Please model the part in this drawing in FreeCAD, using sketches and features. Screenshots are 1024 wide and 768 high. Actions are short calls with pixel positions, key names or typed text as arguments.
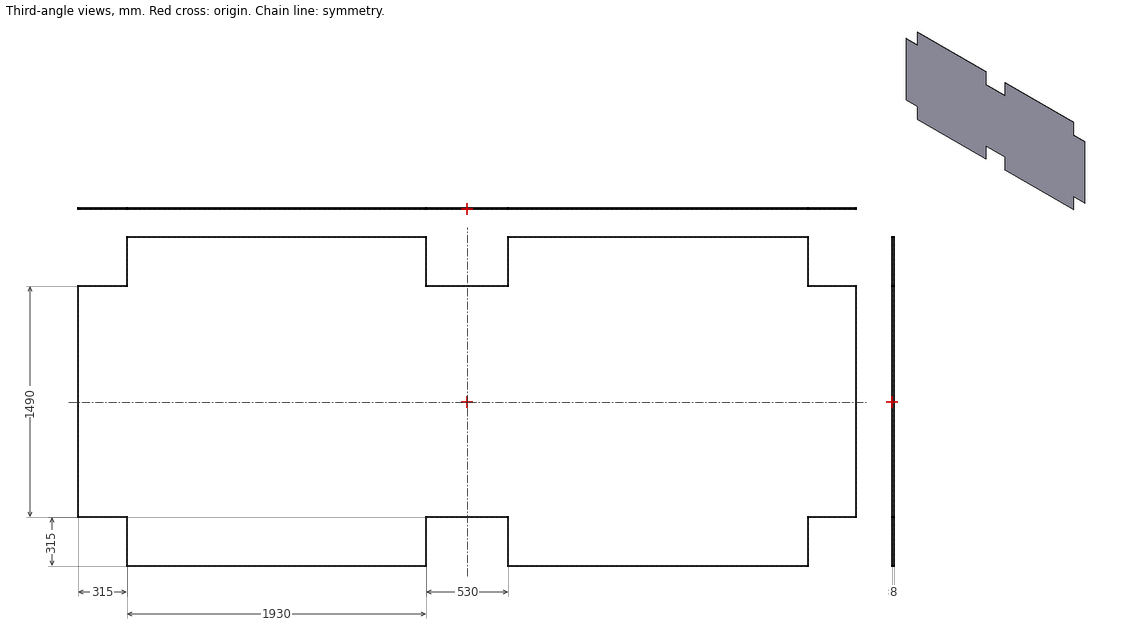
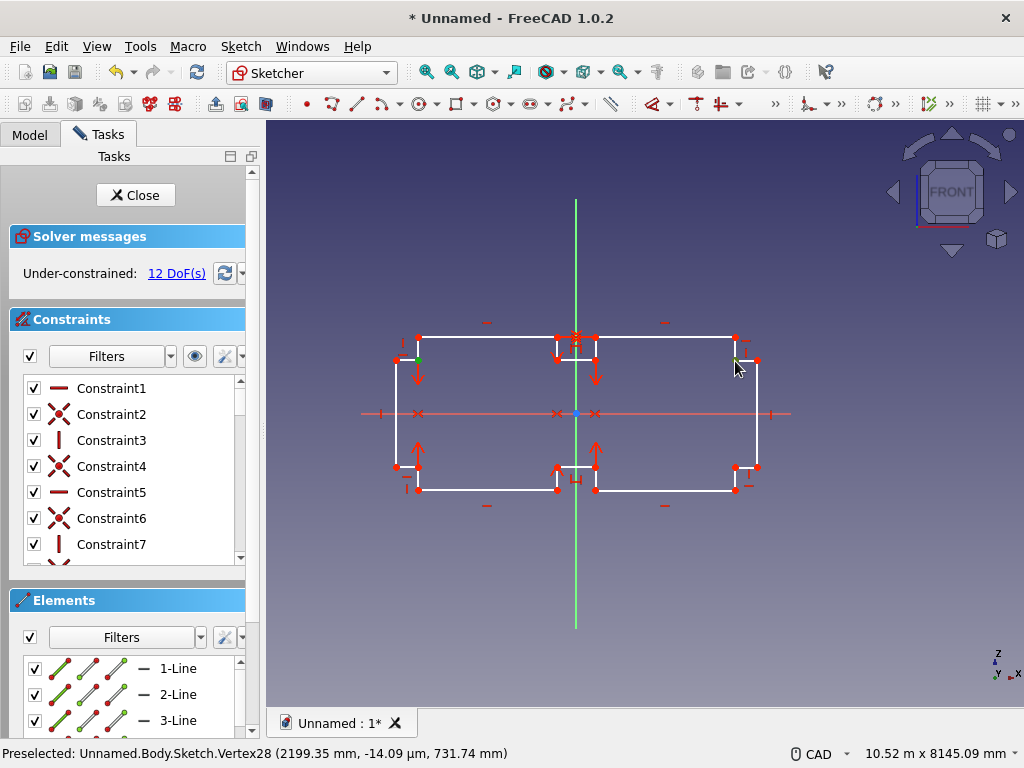
click(576, 603)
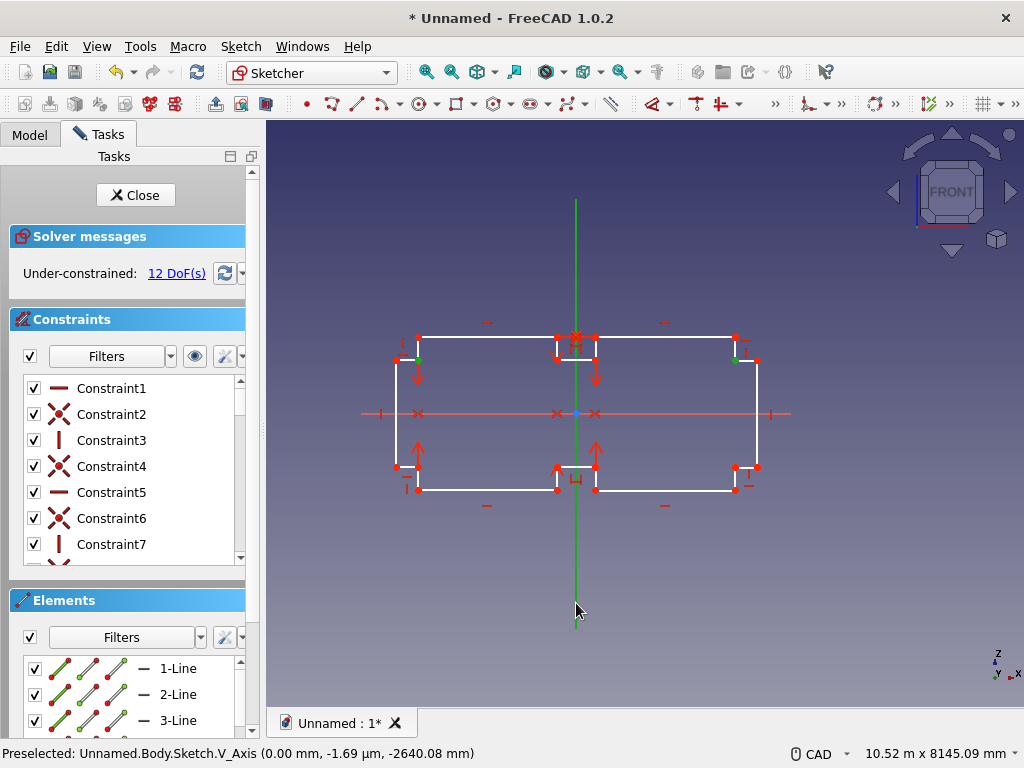
key(s)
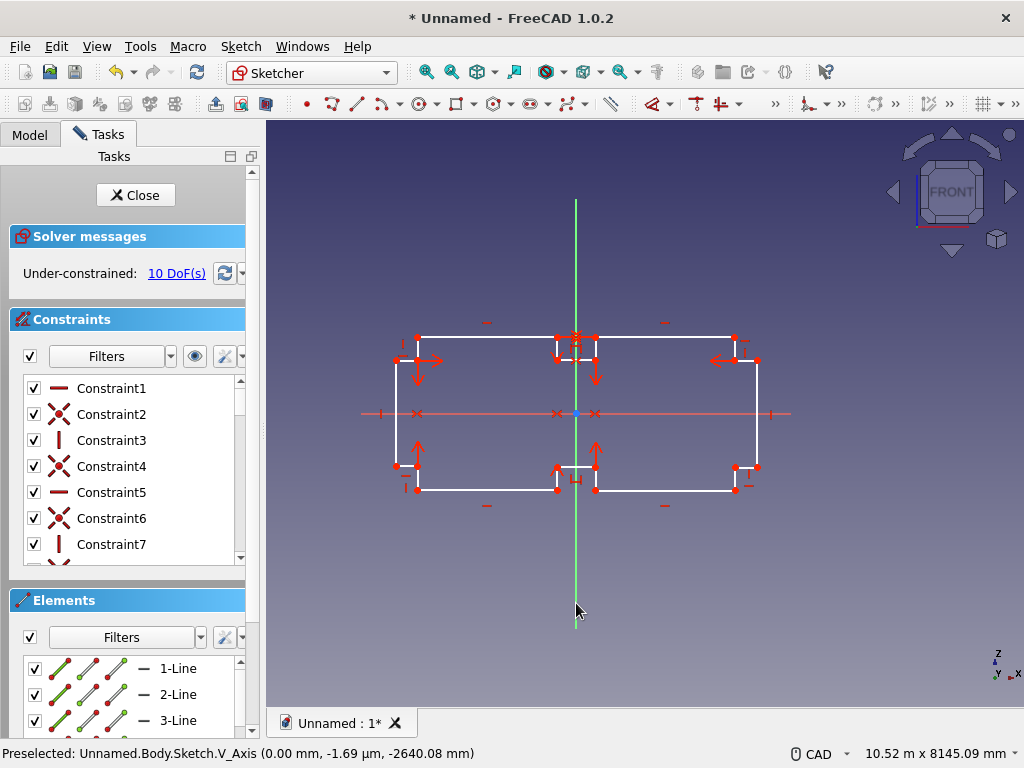
click(396, 466)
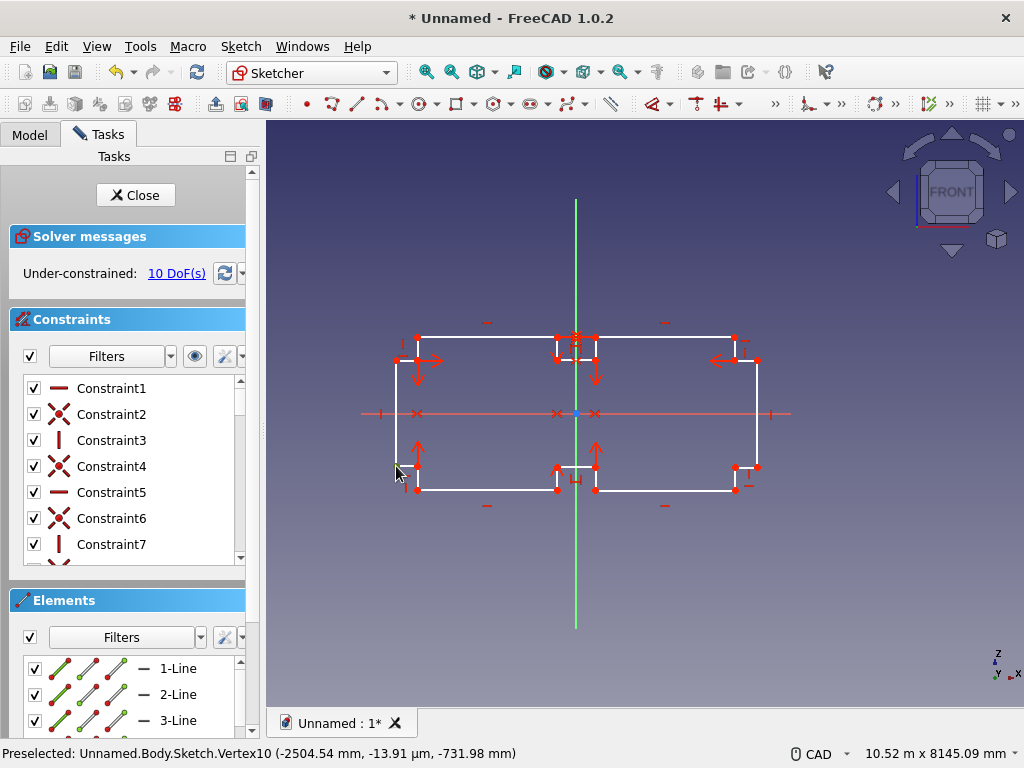
click(757, 468)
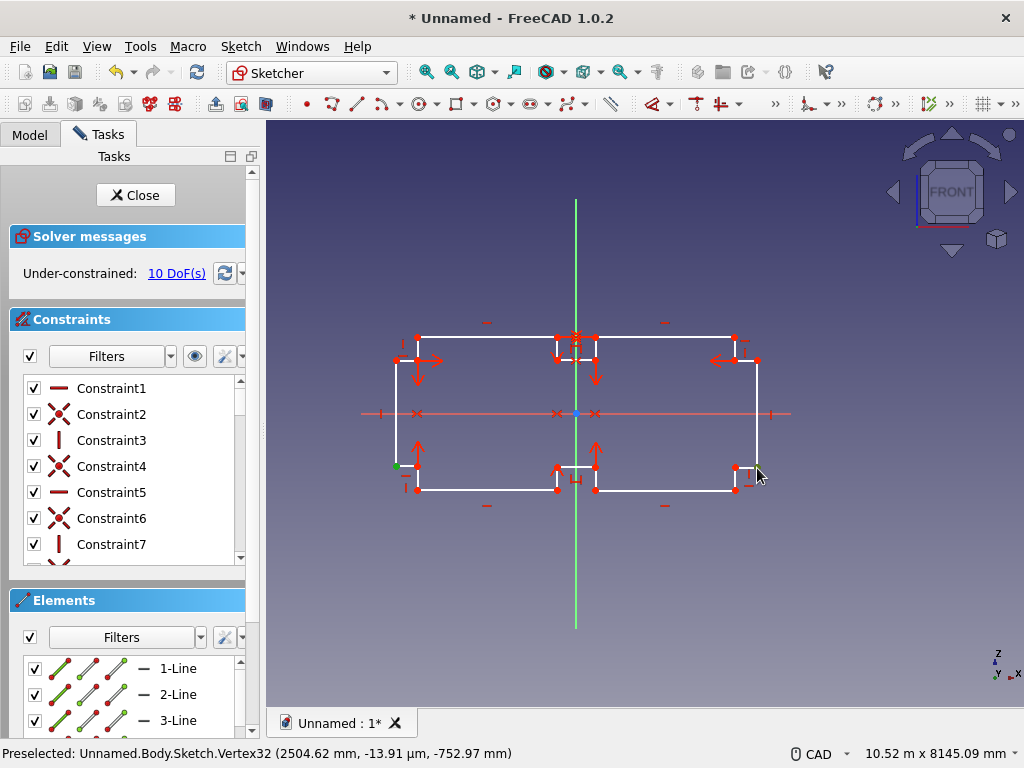
click(576, 603)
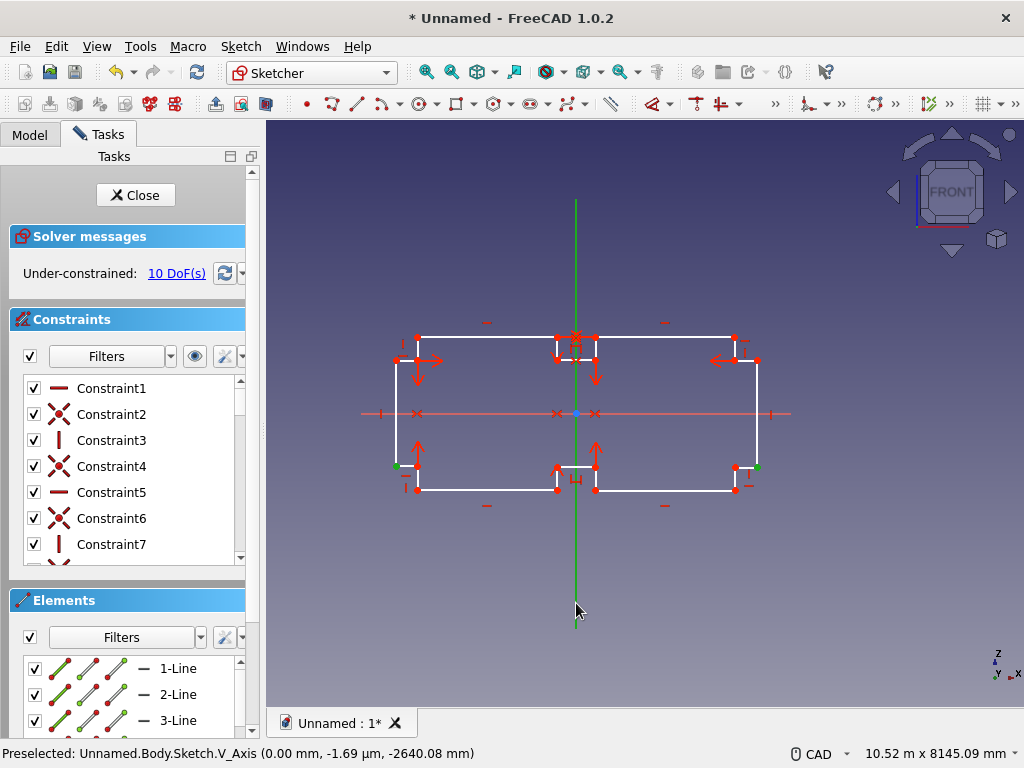
key(s)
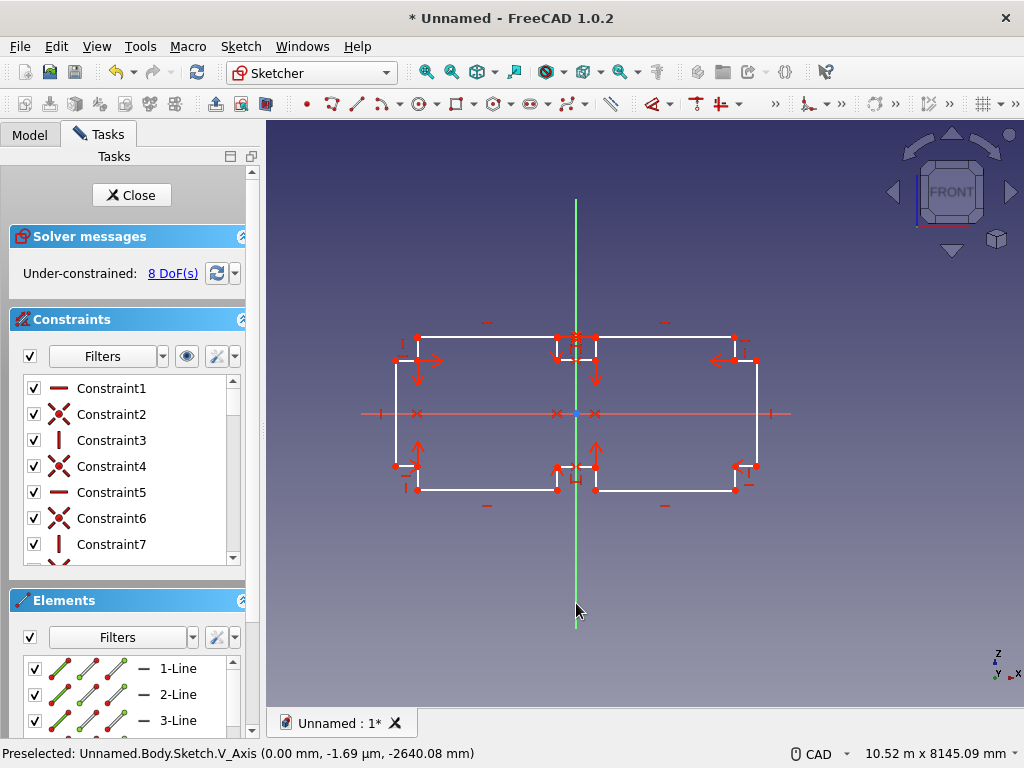
click(418, 490)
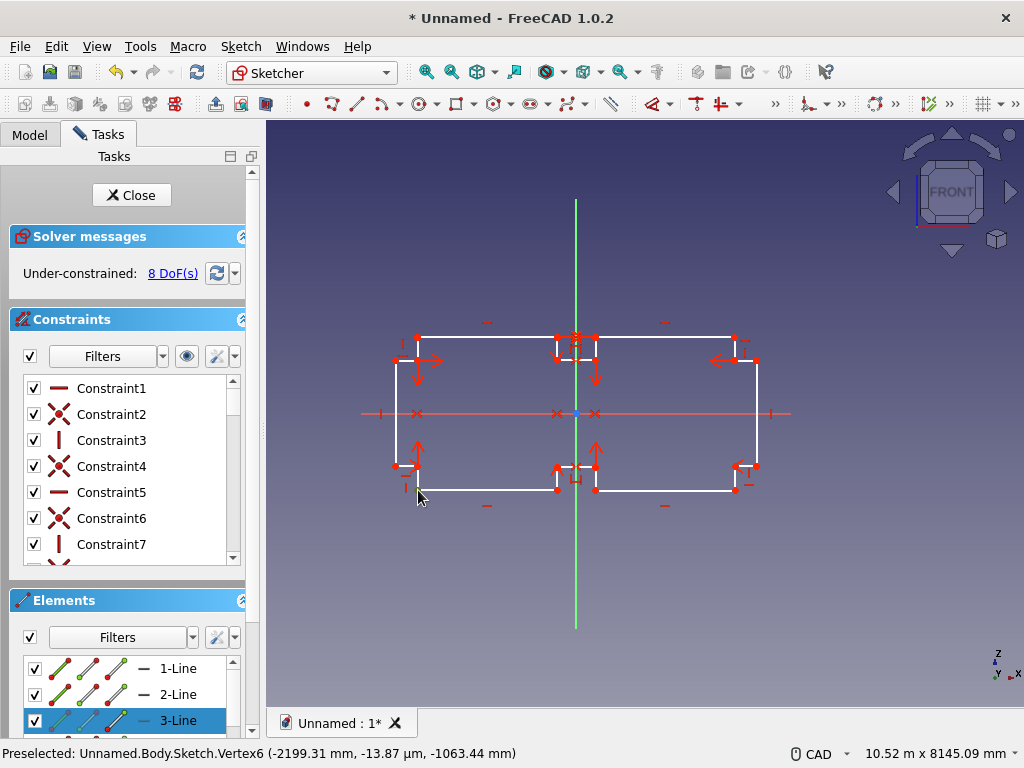
click(735, 491)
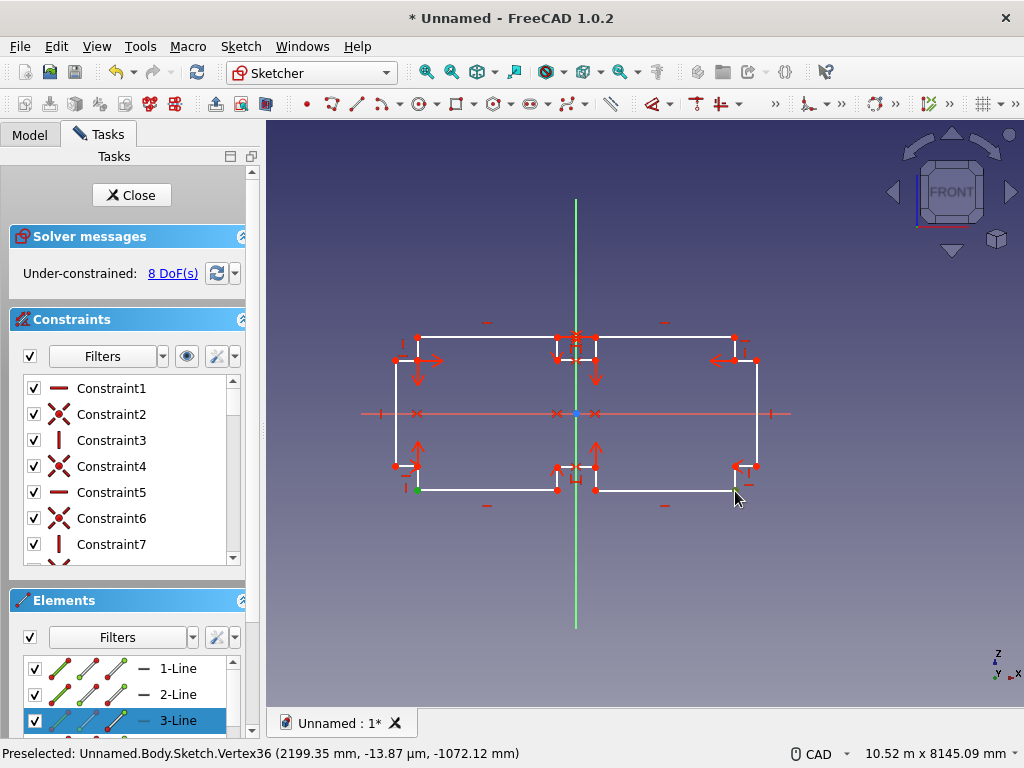
click(576, 603)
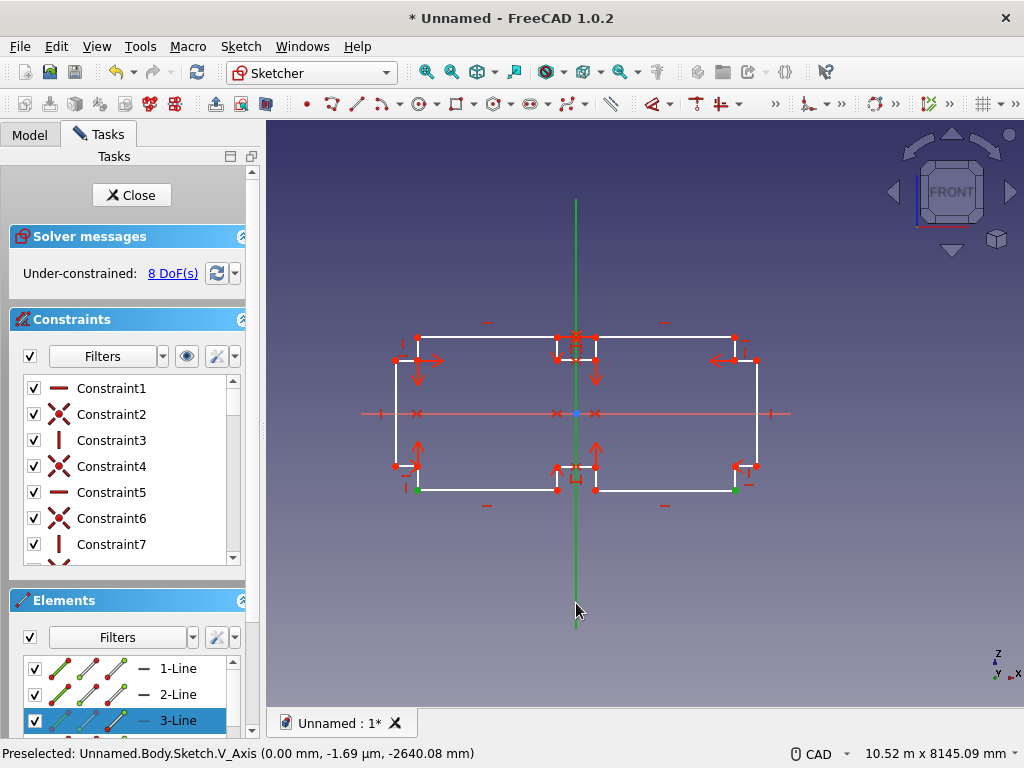
key(s)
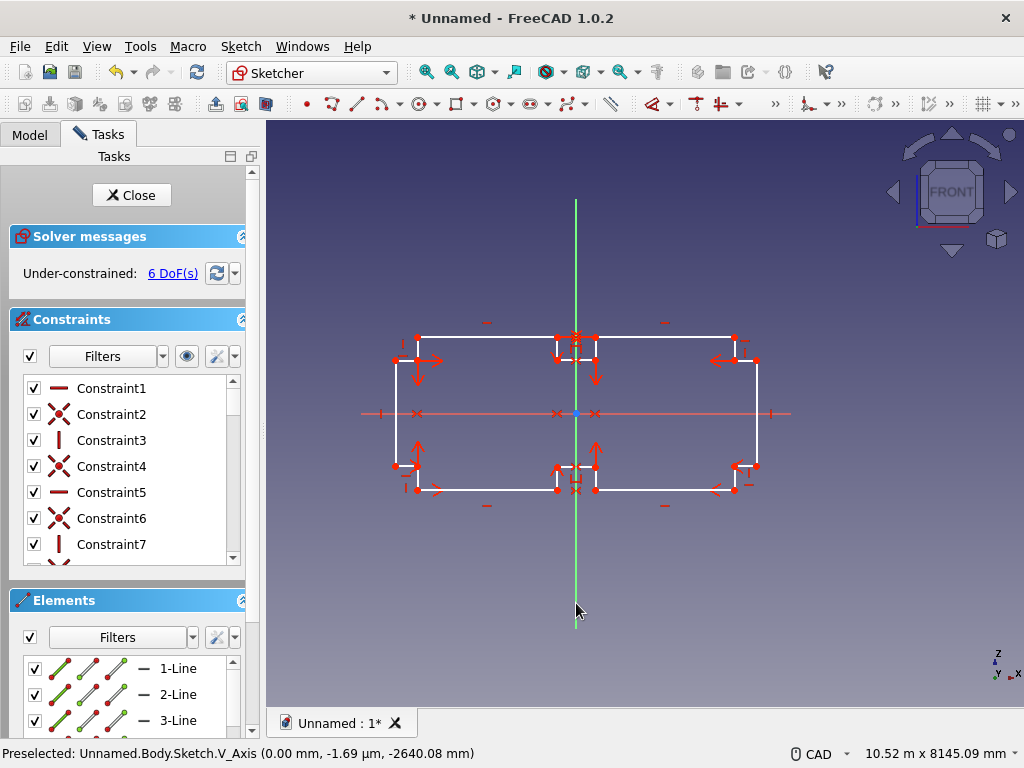
click(652, 104)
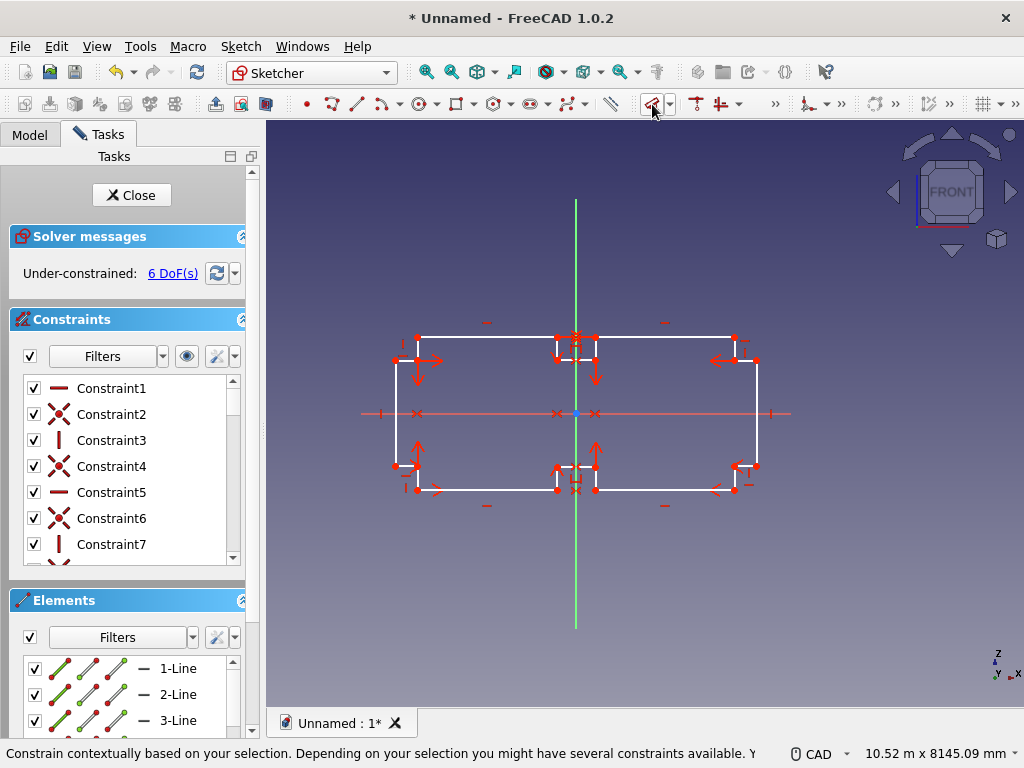
click(580, 467)
click(563, 433)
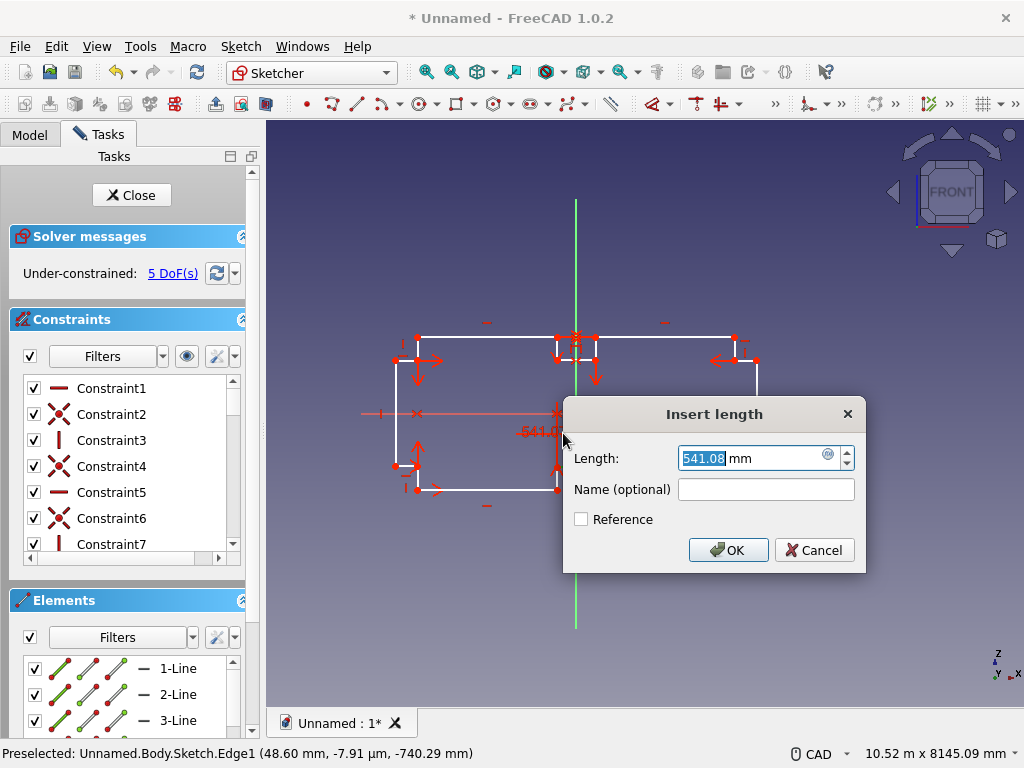
text(530)
key(Return)